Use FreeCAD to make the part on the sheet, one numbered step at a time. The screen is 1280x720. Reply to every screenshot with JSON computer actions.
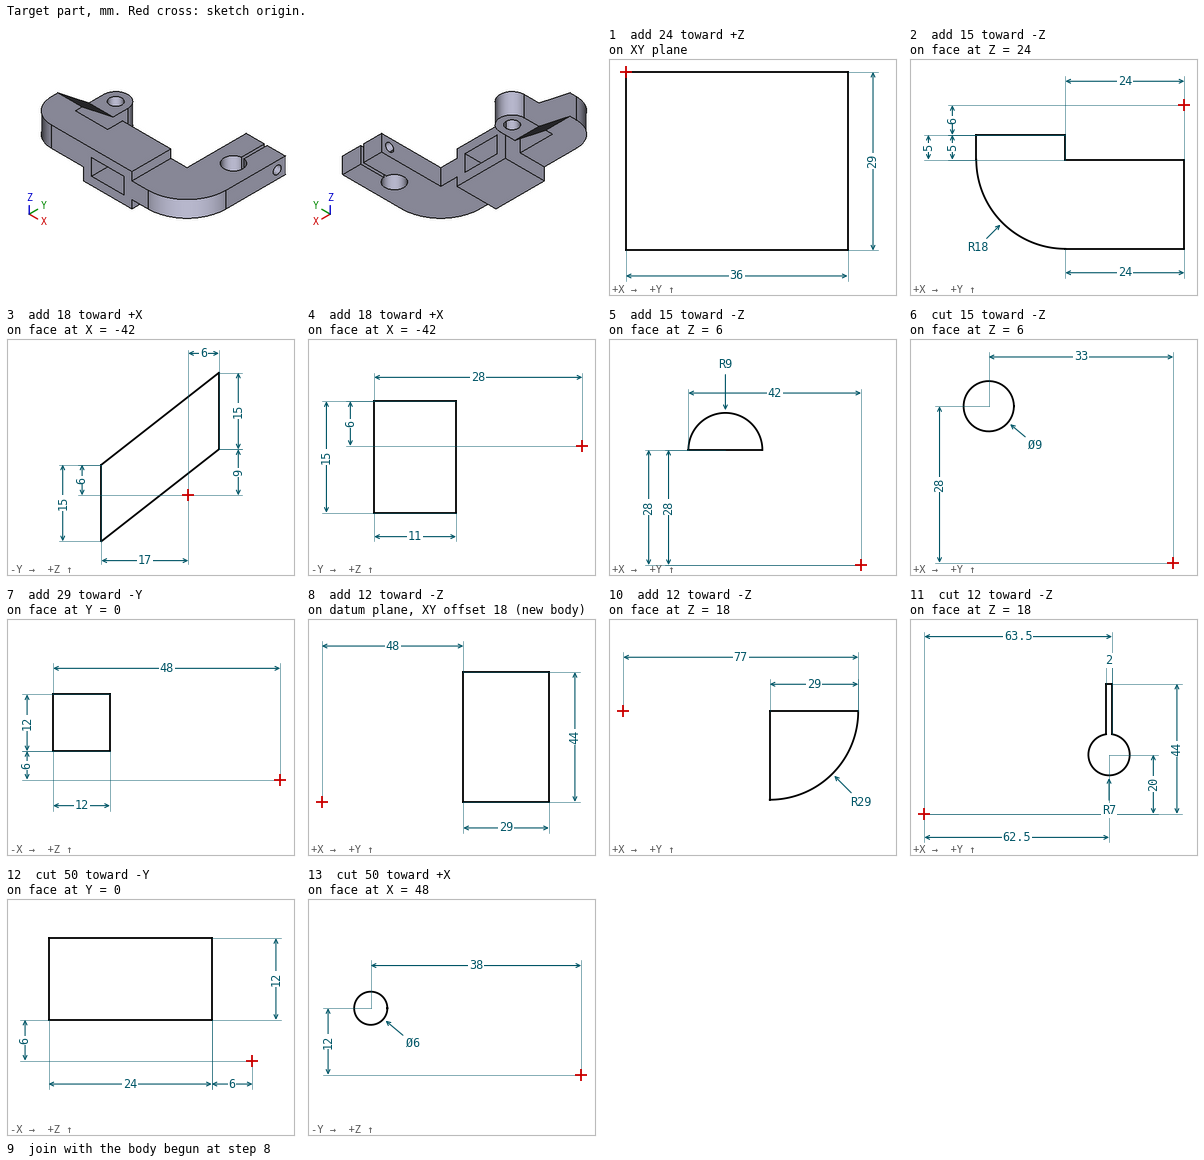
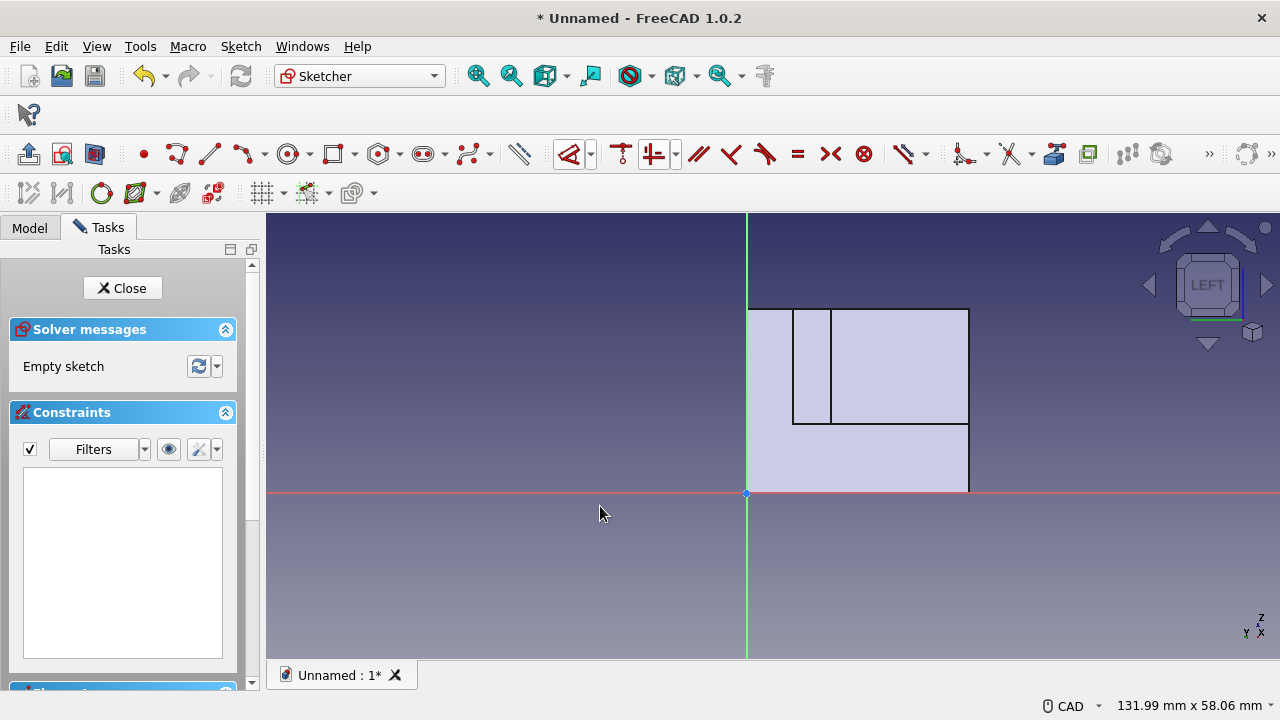
{"action": "left_click", "coordinate": [177, 154]}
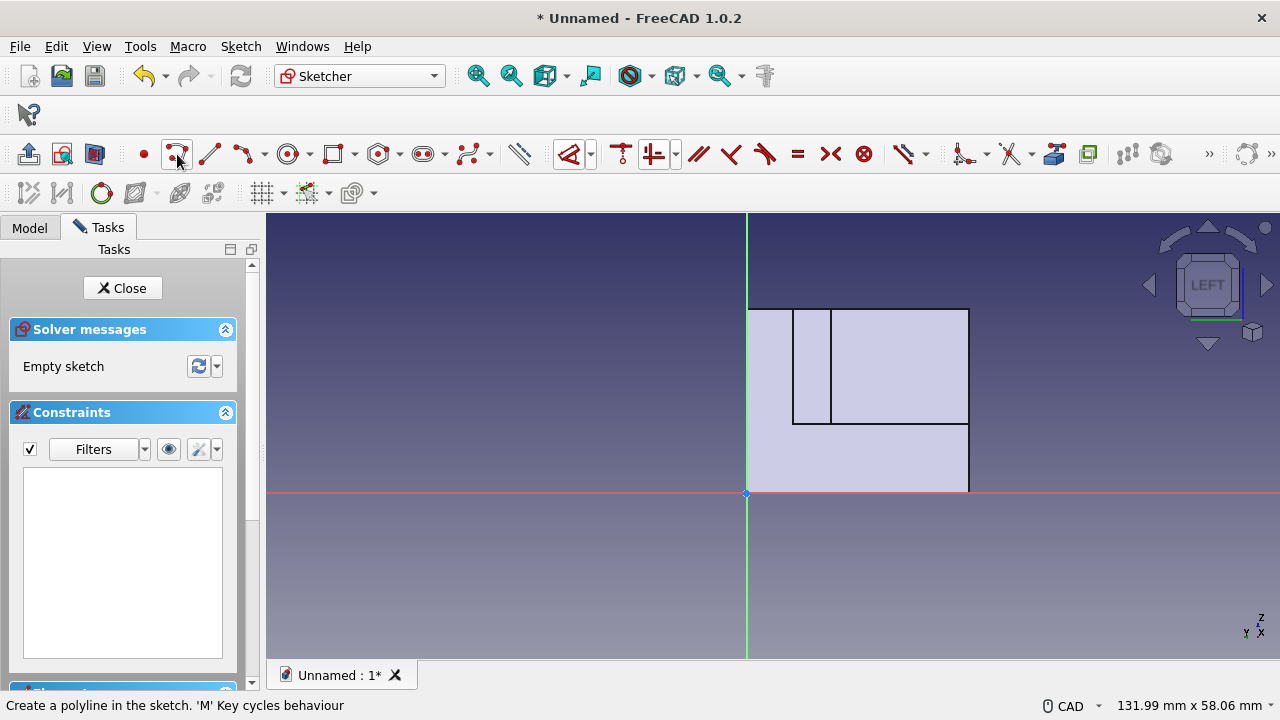
{"action": "left_click", "coordinate": [793, 424]}
{"action": "left_click", "coordinate": [793, 309]}
{"action": "left_click", "coordinate": [616, 447]}
{"action": "left_click", "coordinate": [616, 563]}
{"action": "left_click", "coordinate": [793, 425]}
{"action": "key", "text": "Escape"}
{"action": "key", "text": "Escape"}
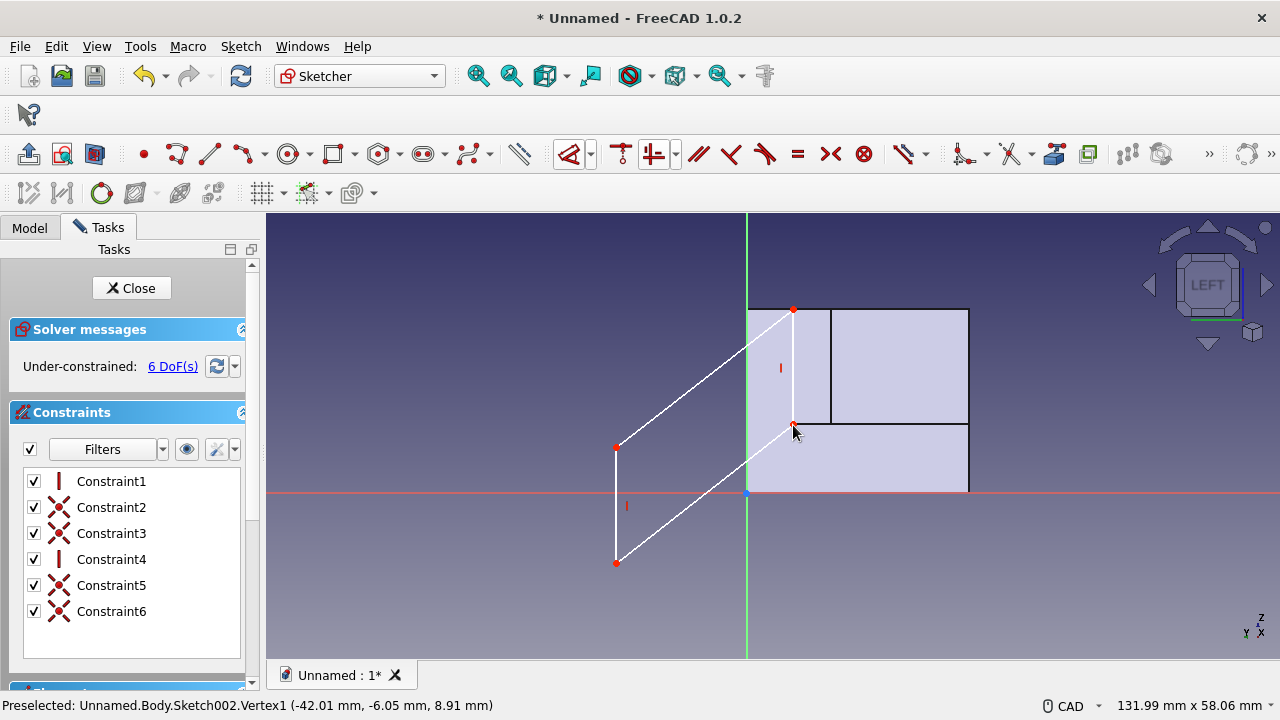
{"action": "left_click", "coordinate": [793, 390]}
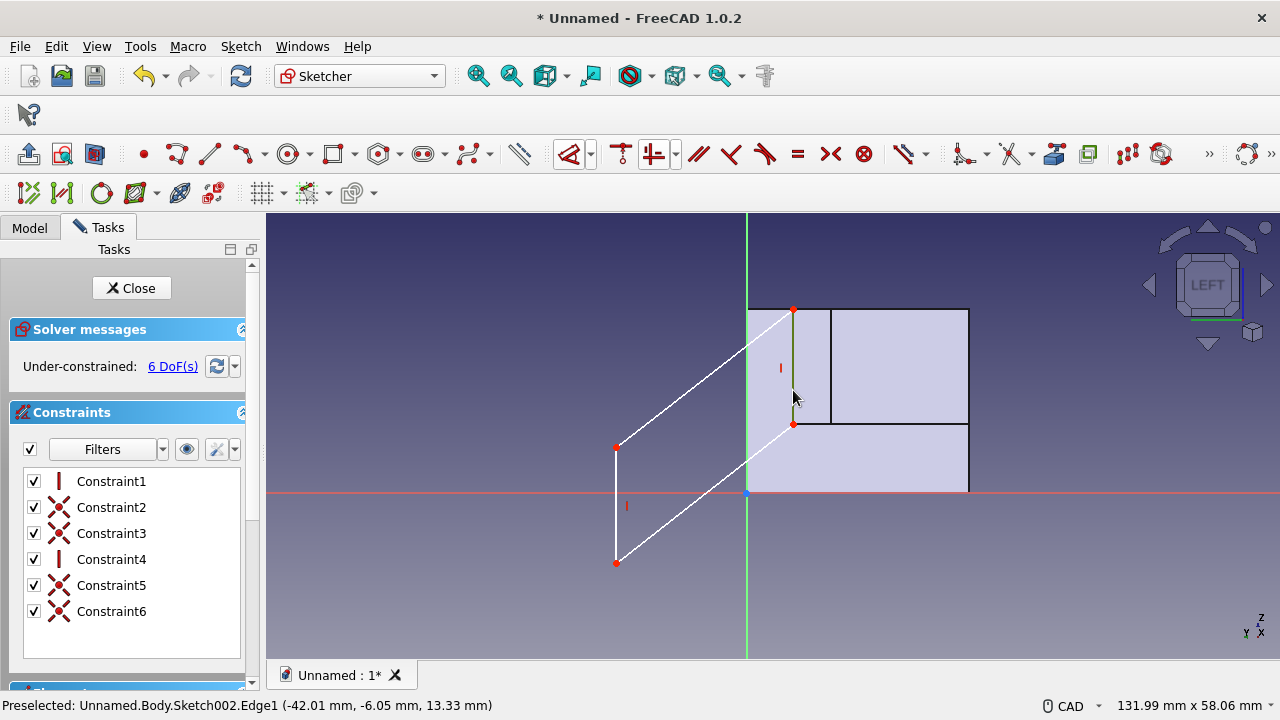
{"action": "key", "text": "i"}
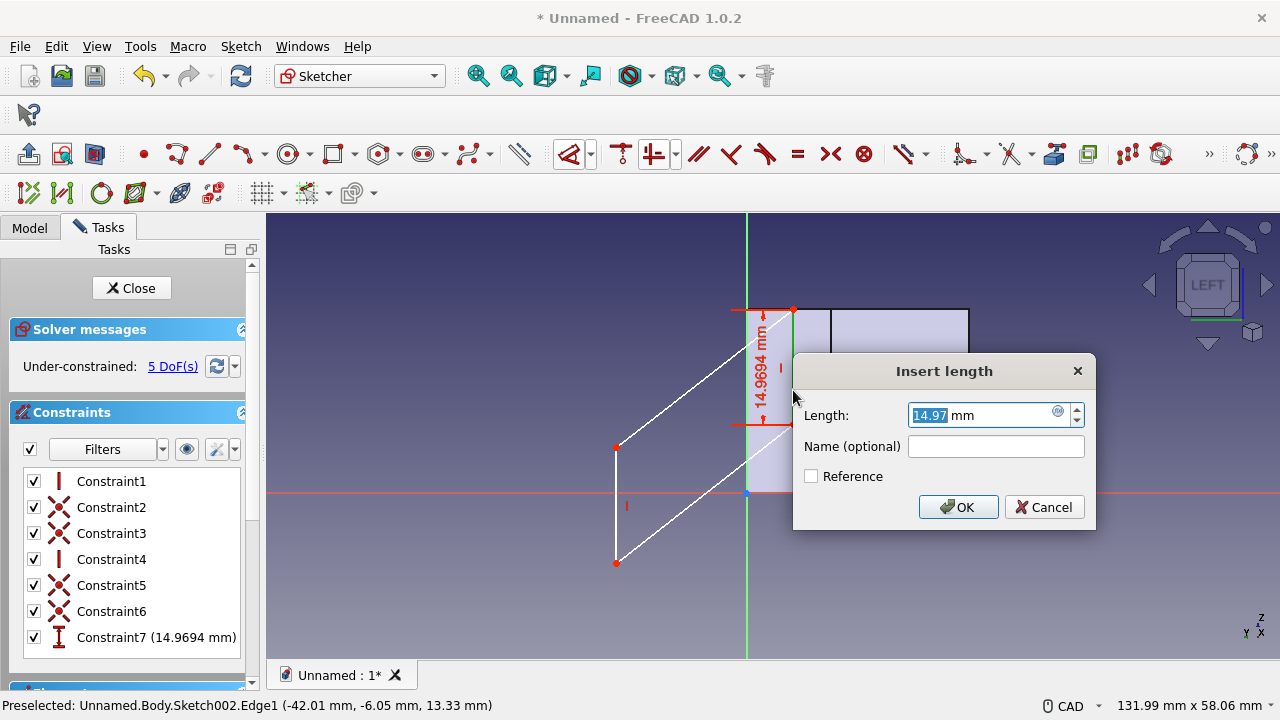
{"action": "type", "text": "15"}
{"action": "key", "text": "Return"}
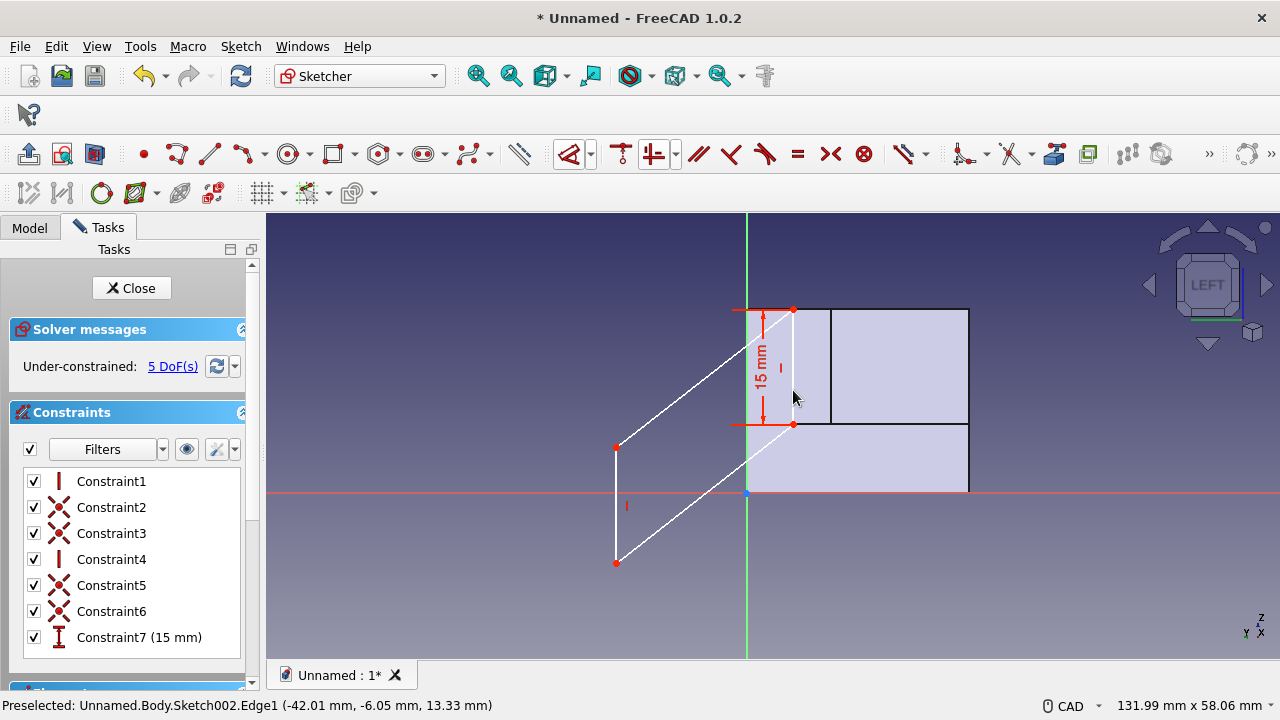
{"action": "scroll", "coordinate": [616, 483], "scroll_direction": "up", "scroll_amount": 2}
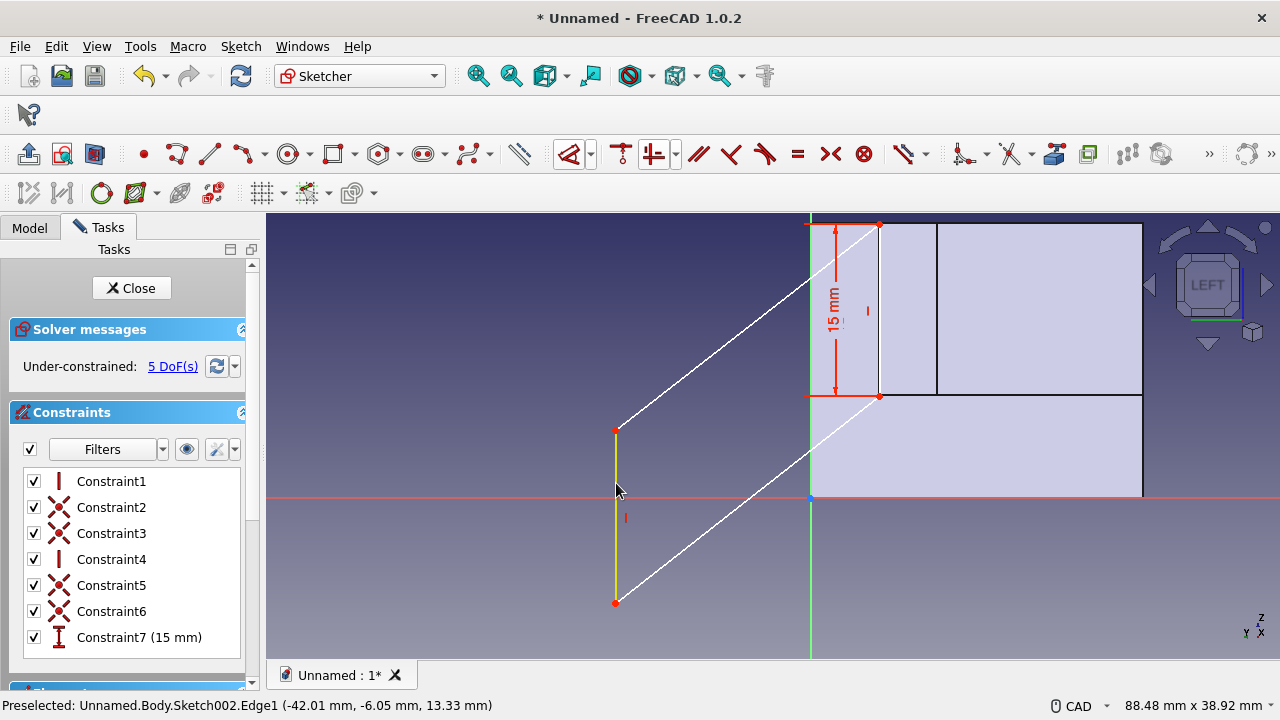
{"action": "left_click", "coordinate": [616, 482]}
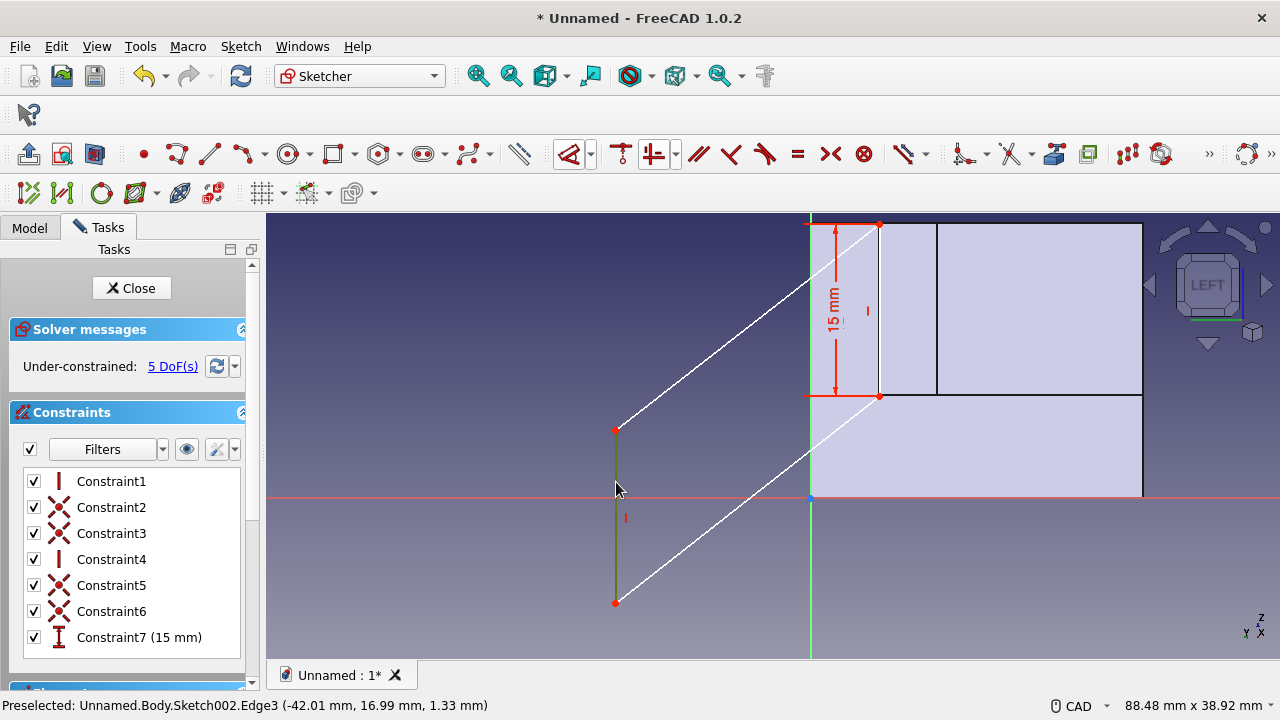
{"action": "key", "text": "i"}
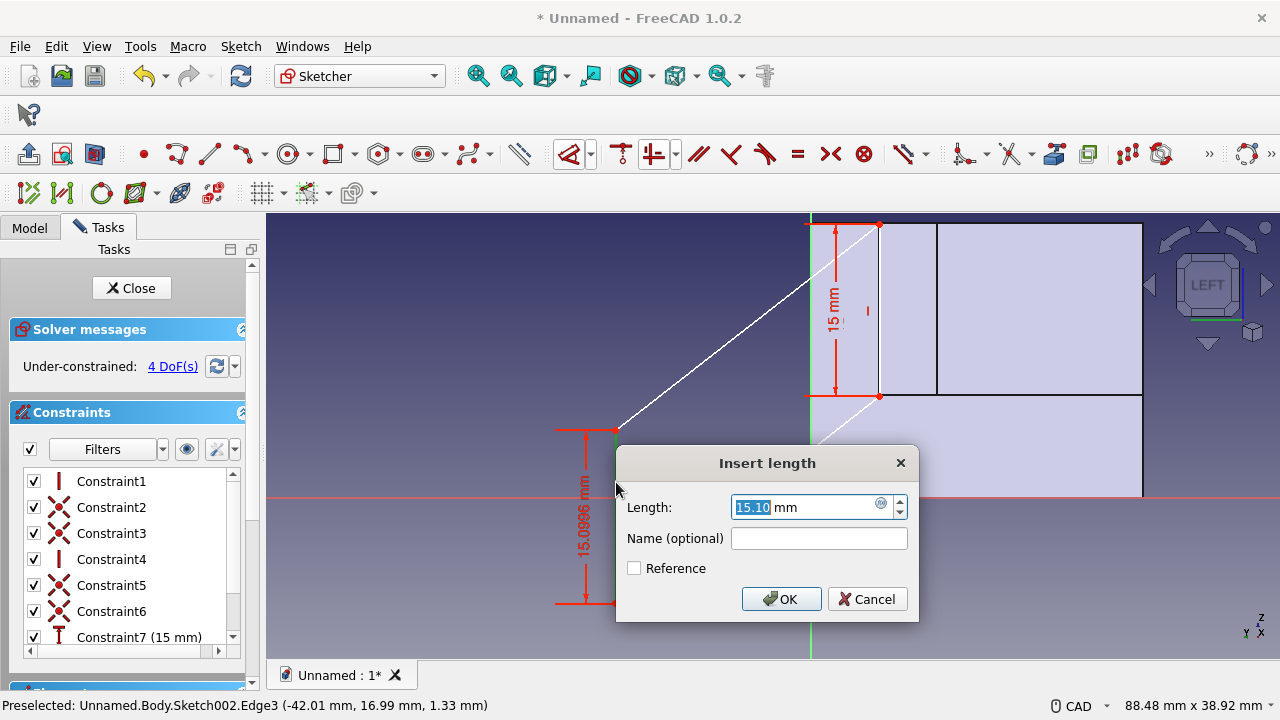
{"action": "type", "text": "15"}
{"action": "key", "text": "Return"}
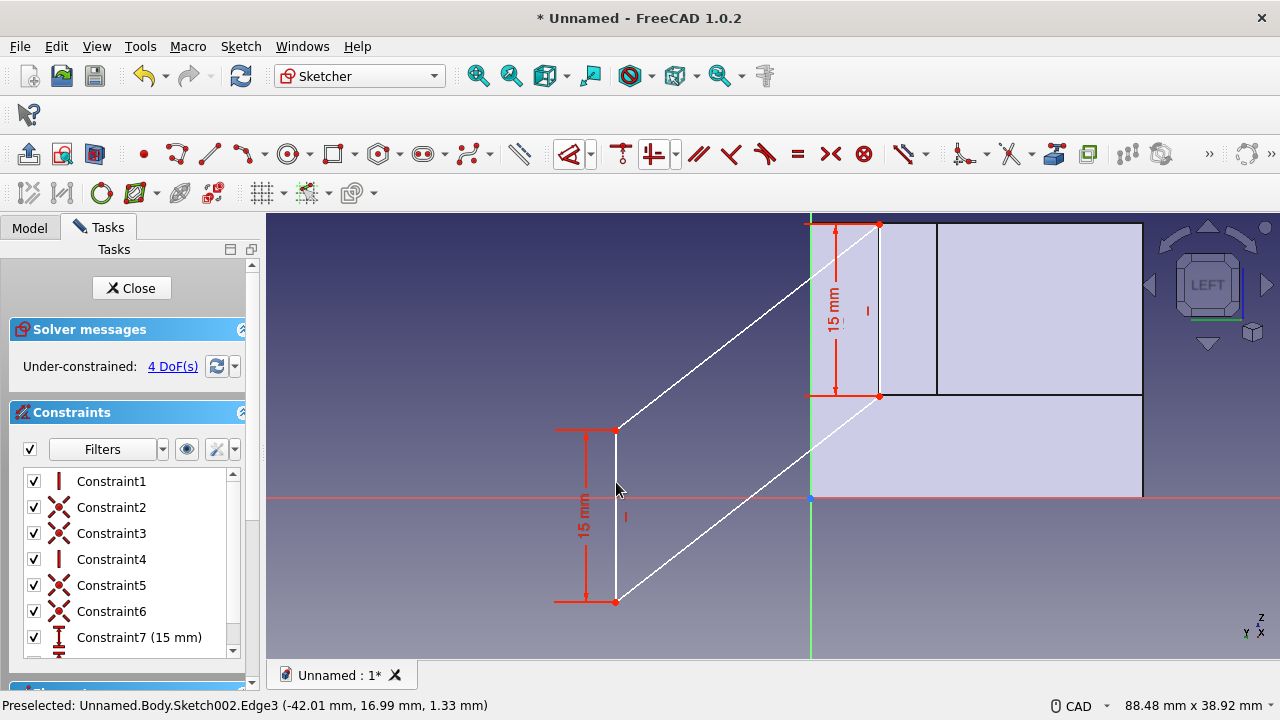
{"action": "left_click", "coordinate": [880, 396]}